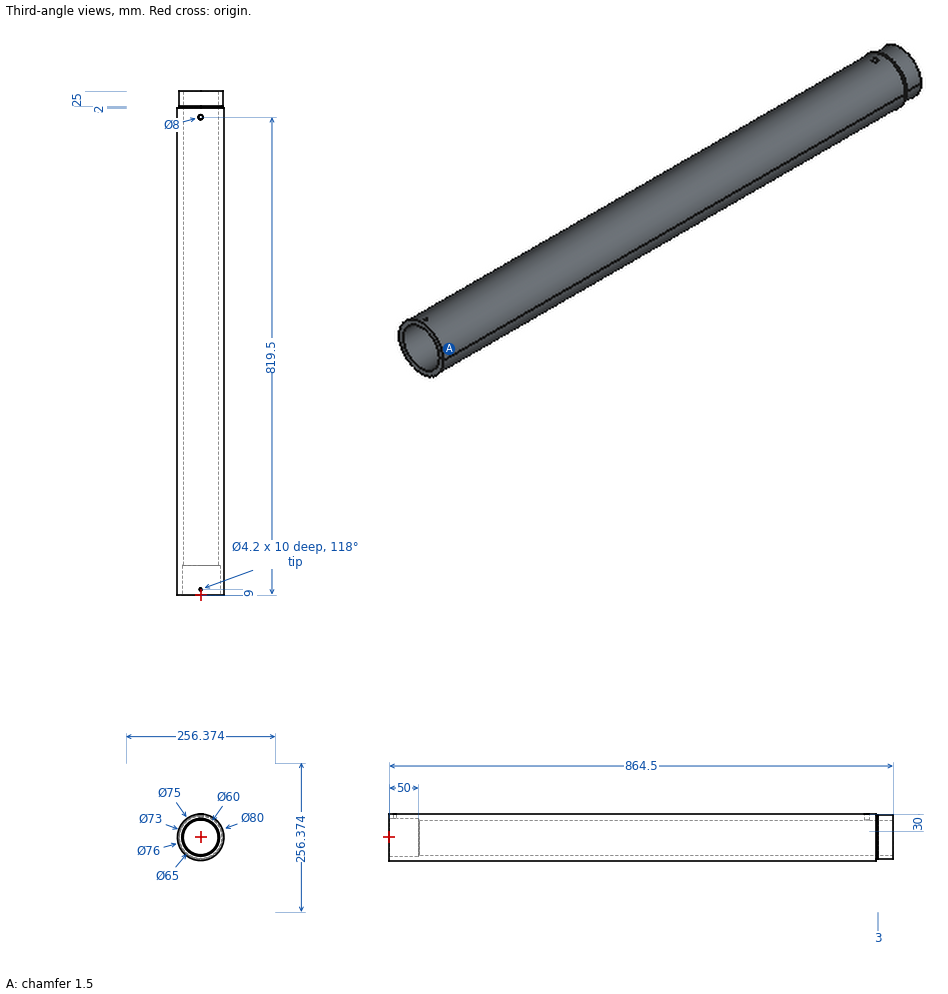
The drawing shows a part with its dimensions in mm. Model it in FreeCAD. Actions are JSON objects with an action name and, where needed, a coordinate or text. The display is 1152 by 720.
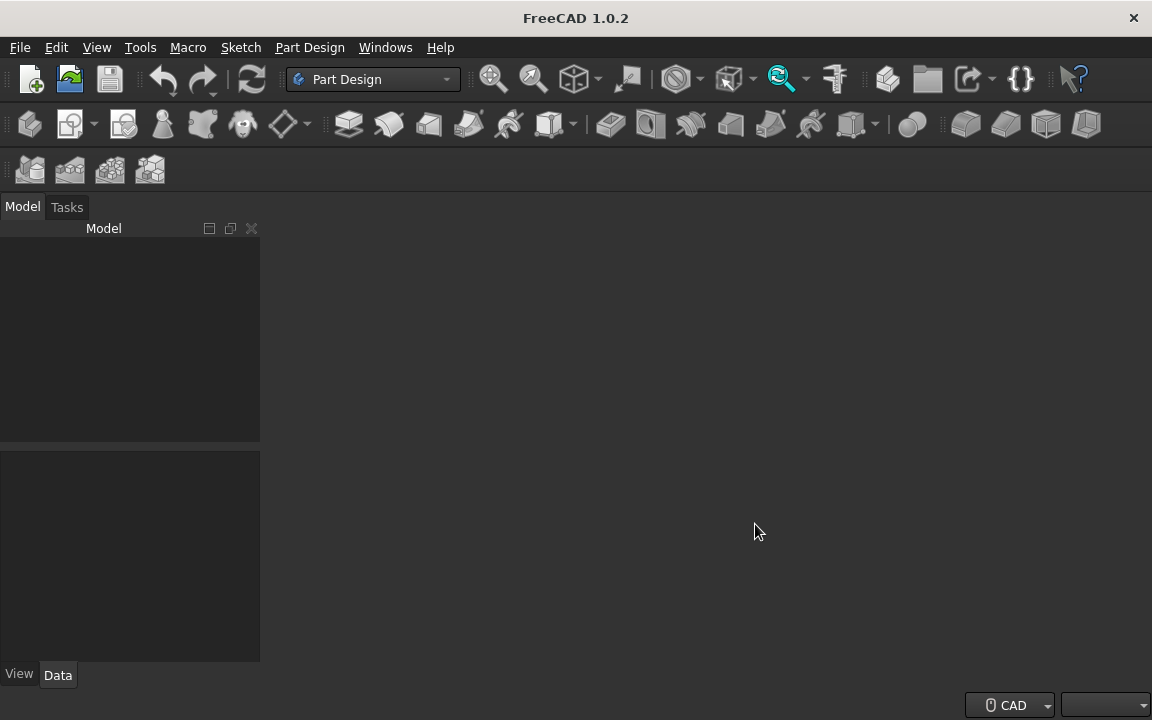
{"action": "left_click", "coordinate": [30, 80]}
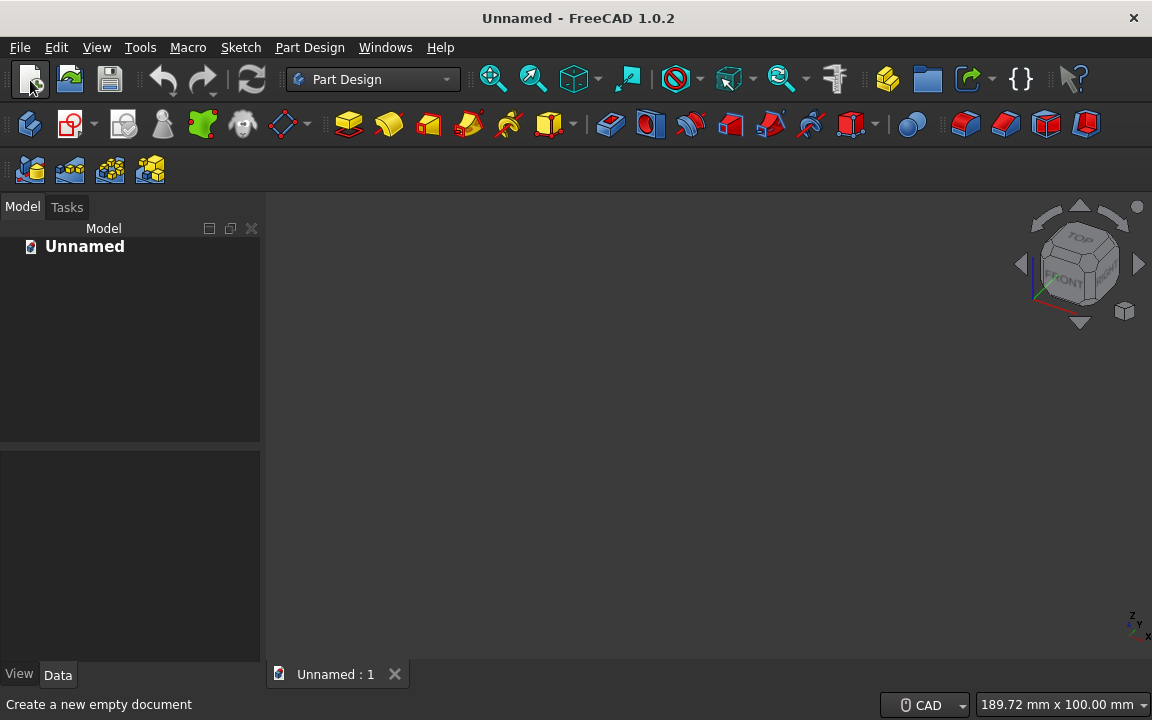
{"action": "left_click", "coordinate": [70, 124]}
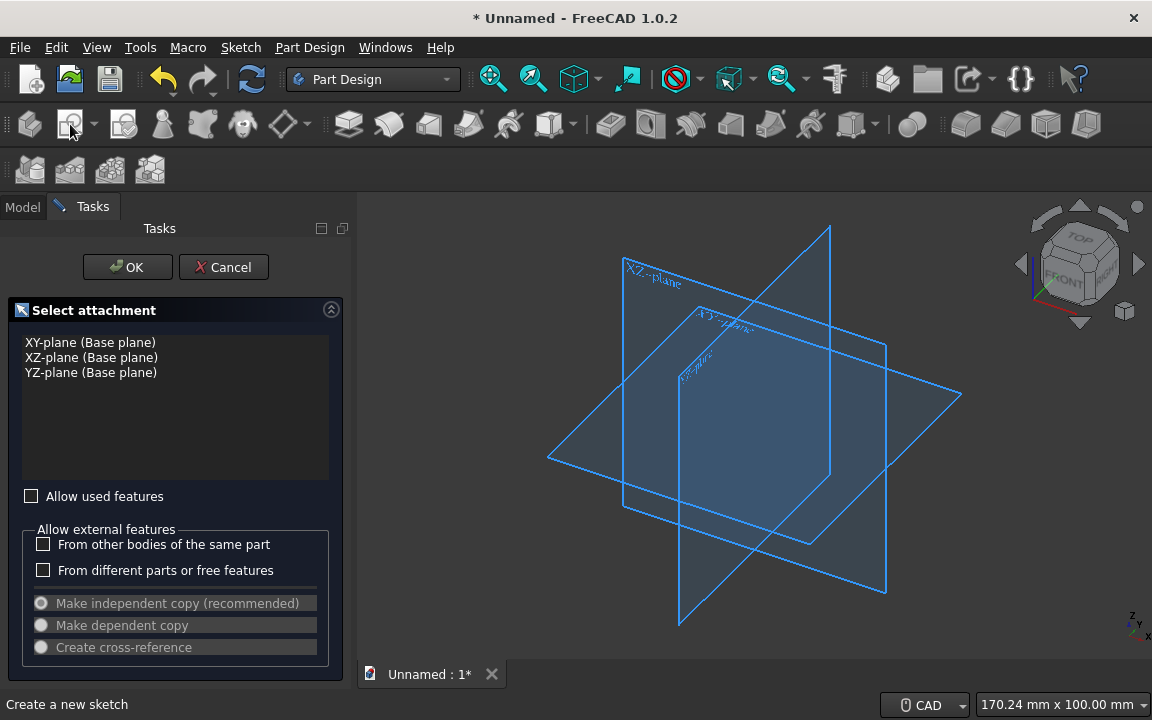
{"action": "left_click", "coordinate": [82, 358]}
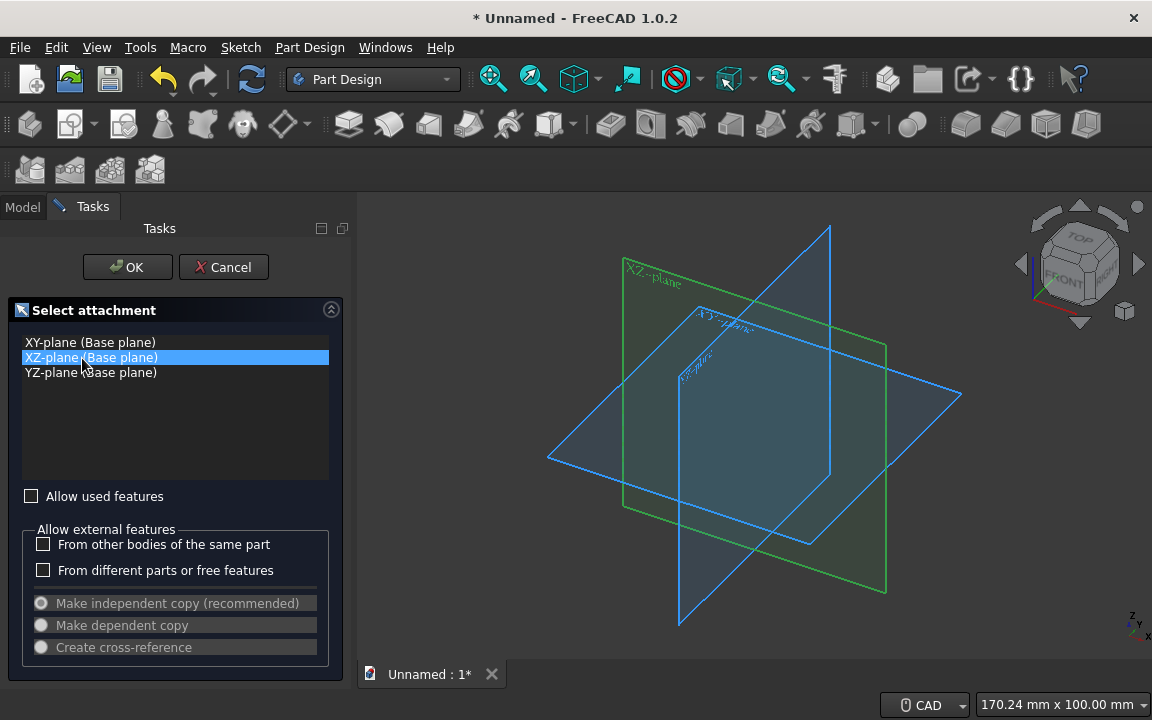
{"action": "left_click", "coordinate": [128, 267]}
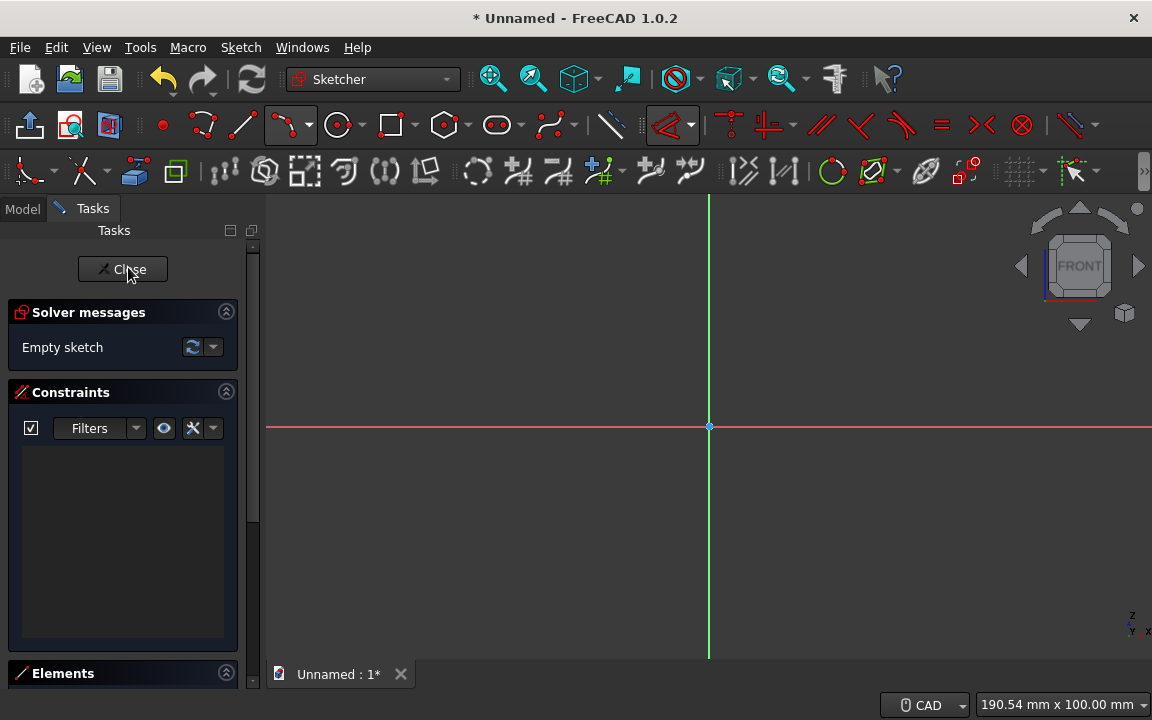
{"action": "scroll", "coordinate": [331, 427], "scroll_direction": "down", "scroll_amount": 1}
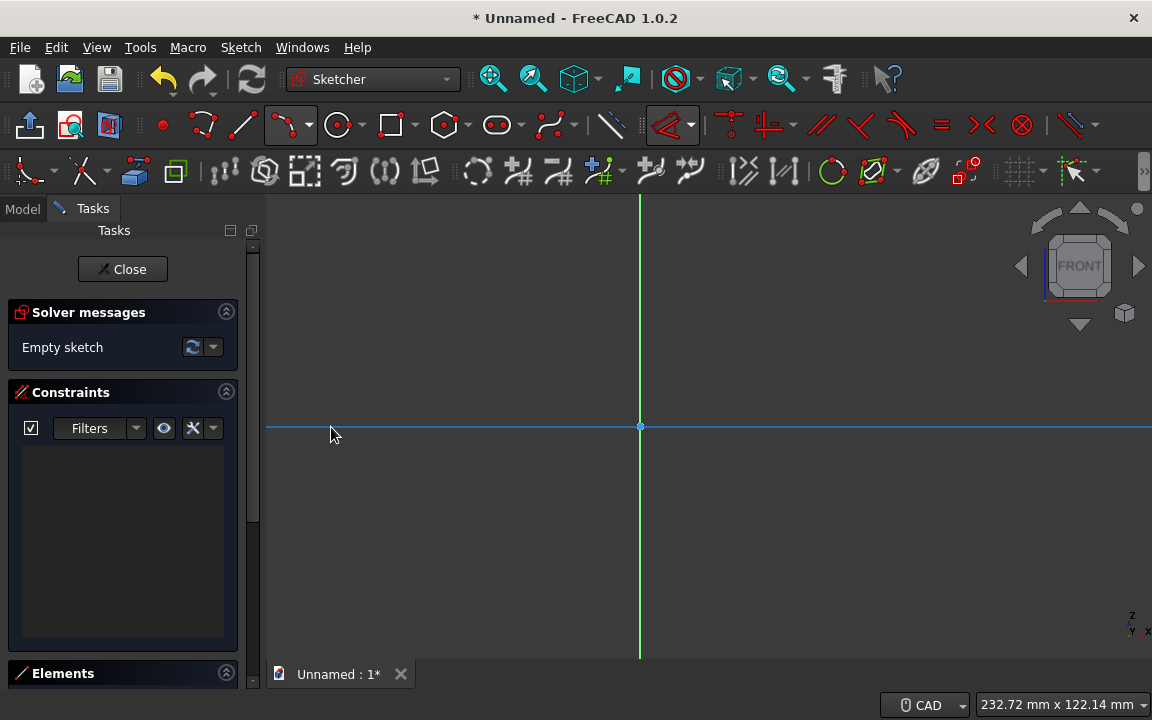
{"action": "left_click", "coordinate": [338, 126]}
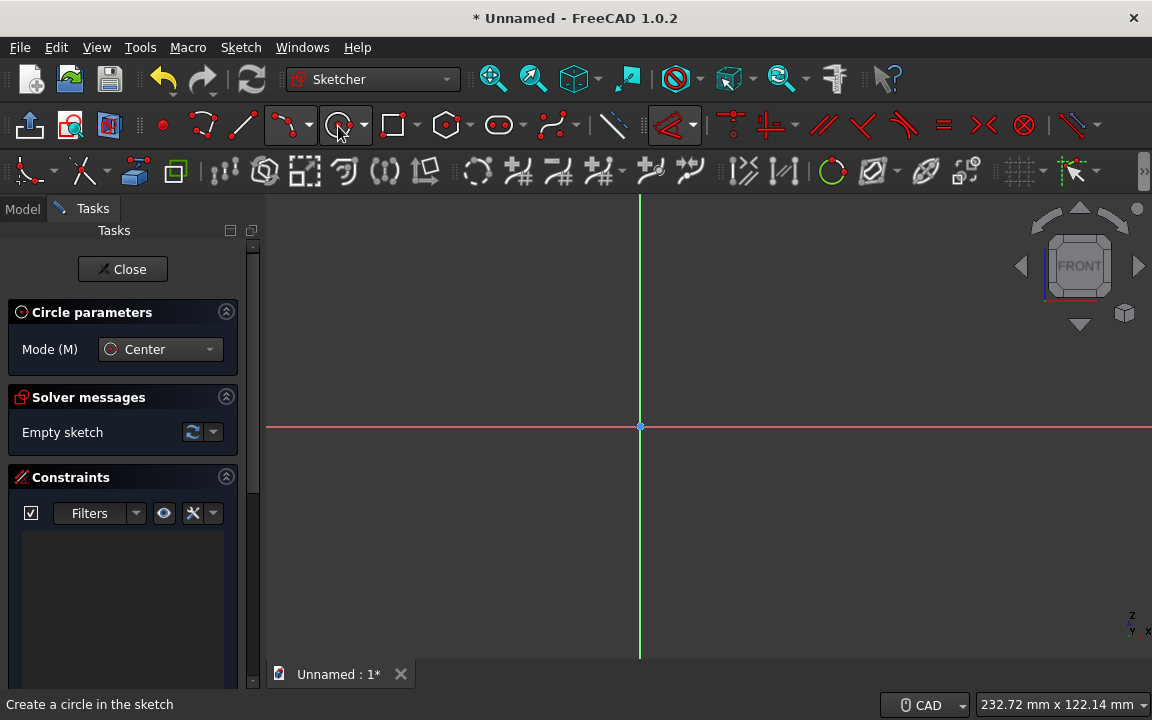
{"action": "left_click", "coordinate": [640, 427]}
{"action": "mouse_move", "coordinate": [748, 319]}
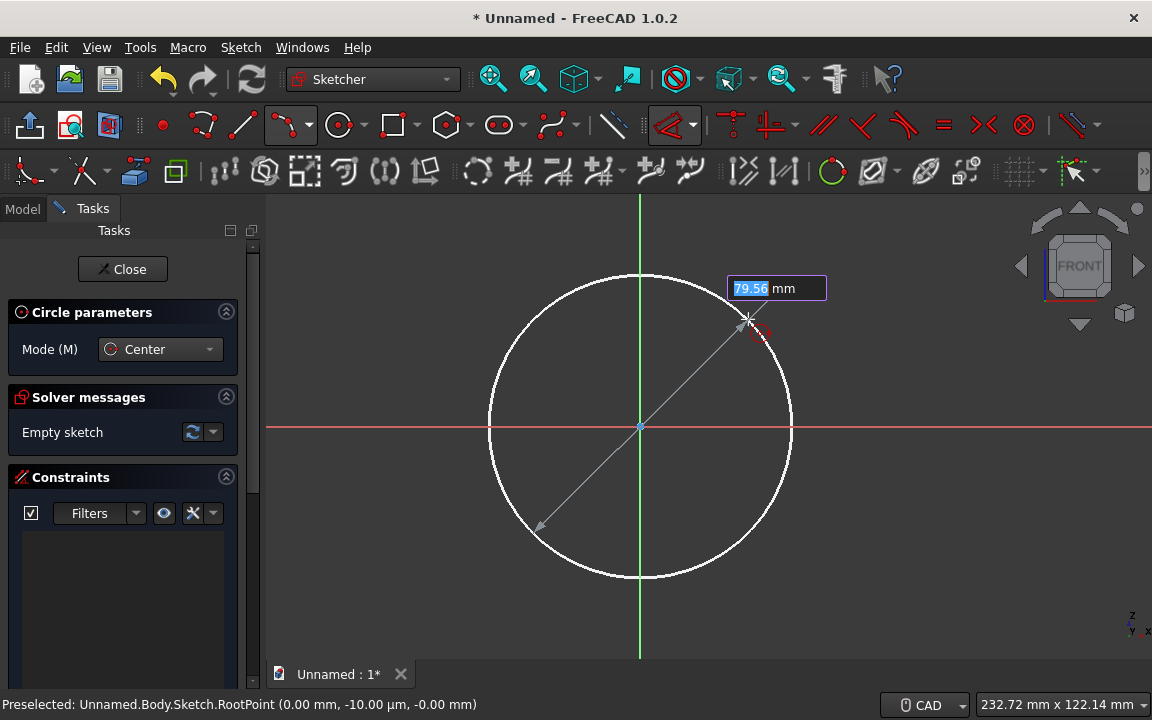
{"action": "type", "text": "80"}
{"action": "key", "text": "Return"}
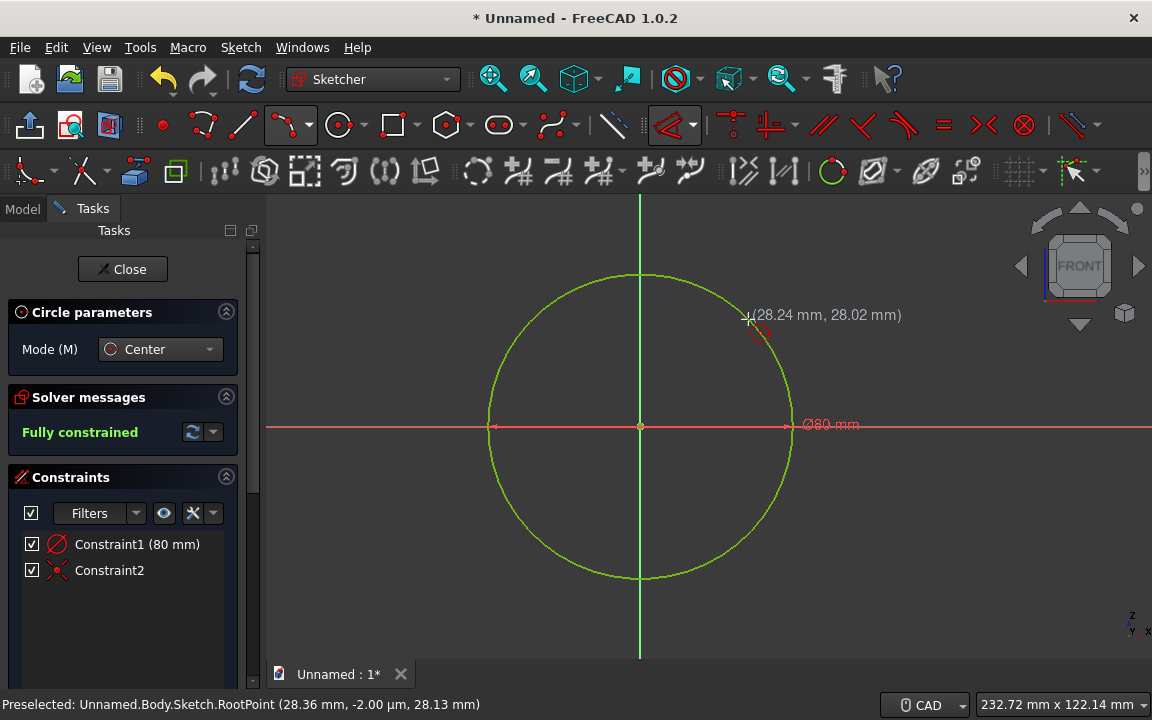
{"action": "left_click", "coordinate": [640, 427]}
{"action": "mouse_move", "coordinate": [721, 346]}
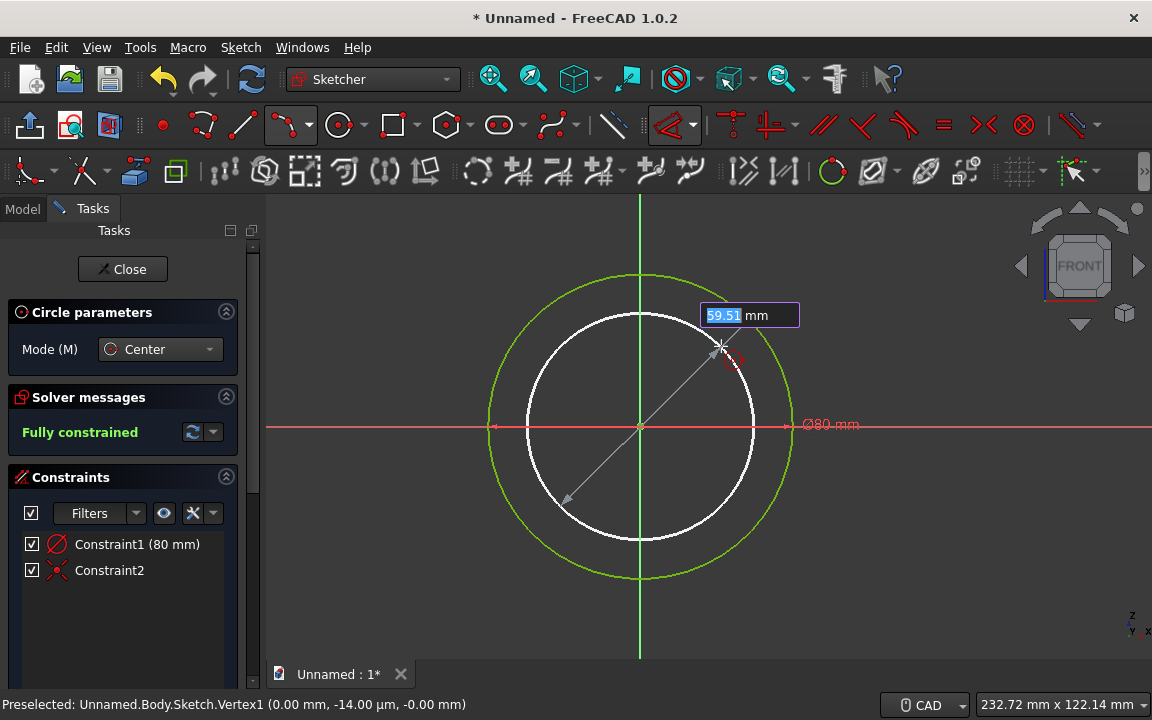
{"action": "type", "text": "60"}
{"action": "key", "text": "Return"}
{"action": "key", "text": "Escape"}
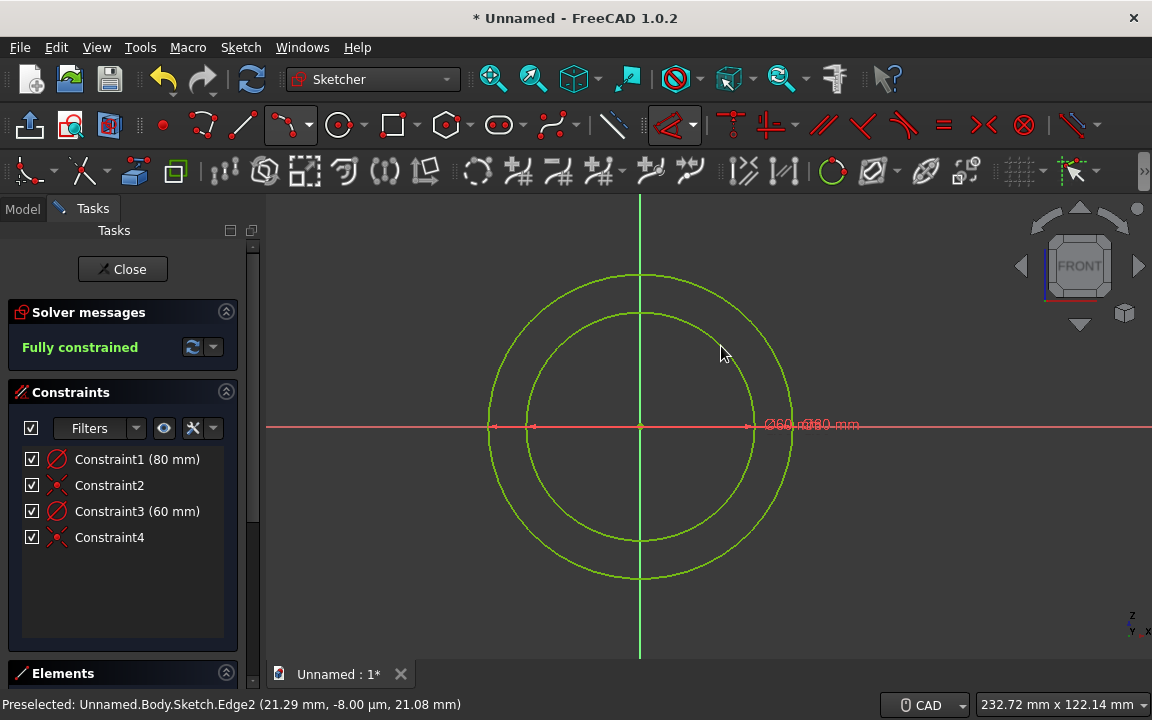
{"action": "left_click", "coordinate": [123, 269]}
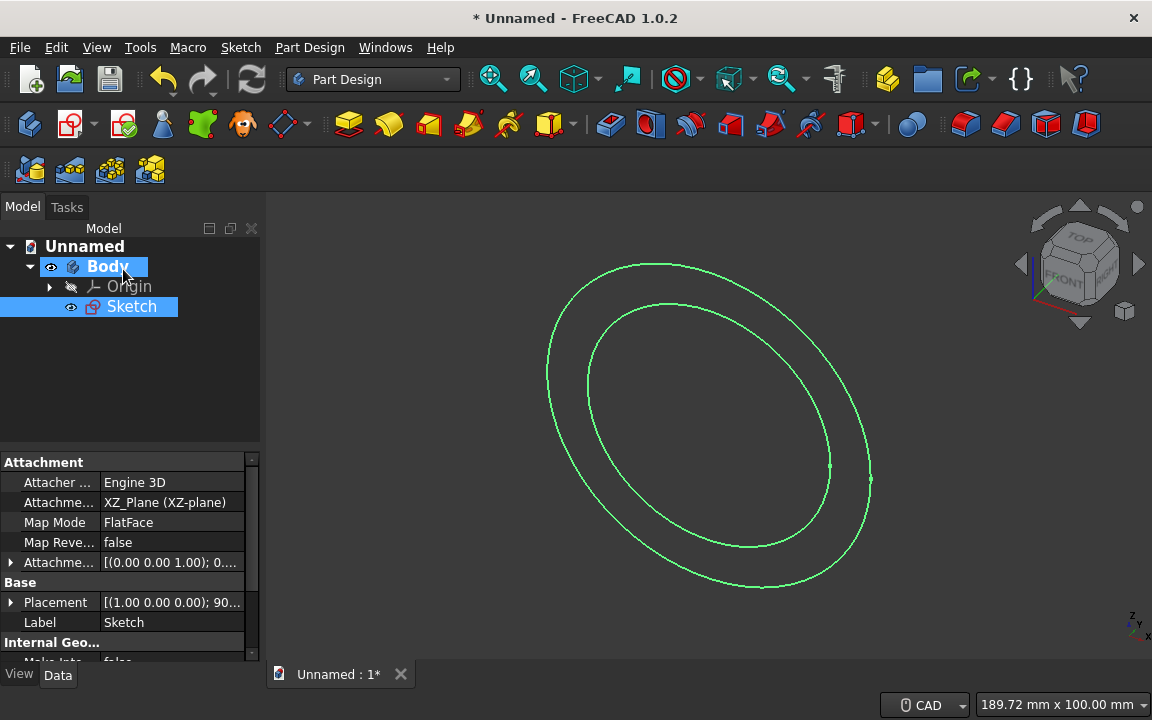
{"action": "left_click", "coordinate": [350, 124]}